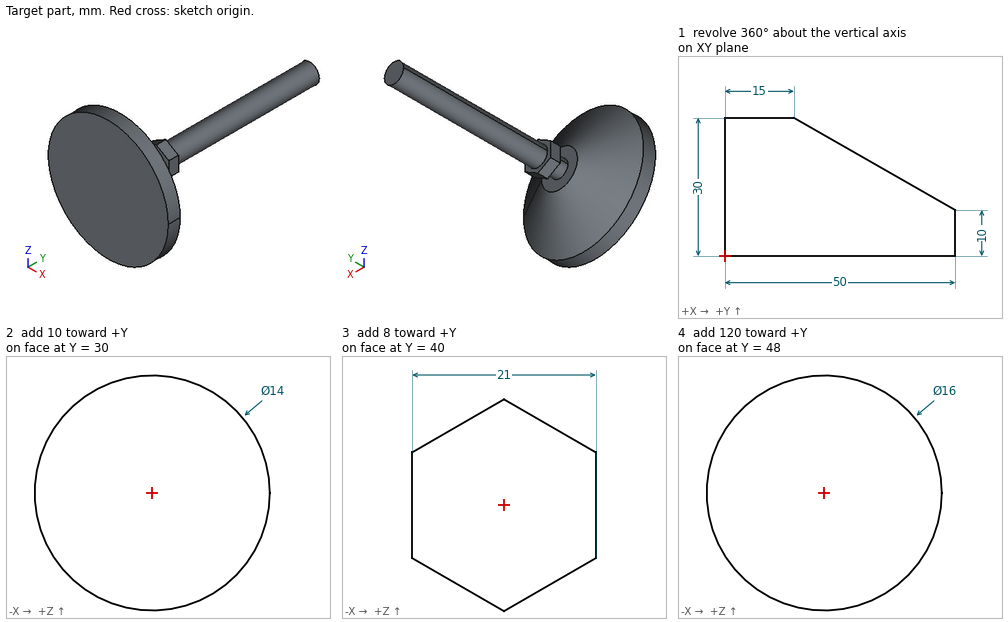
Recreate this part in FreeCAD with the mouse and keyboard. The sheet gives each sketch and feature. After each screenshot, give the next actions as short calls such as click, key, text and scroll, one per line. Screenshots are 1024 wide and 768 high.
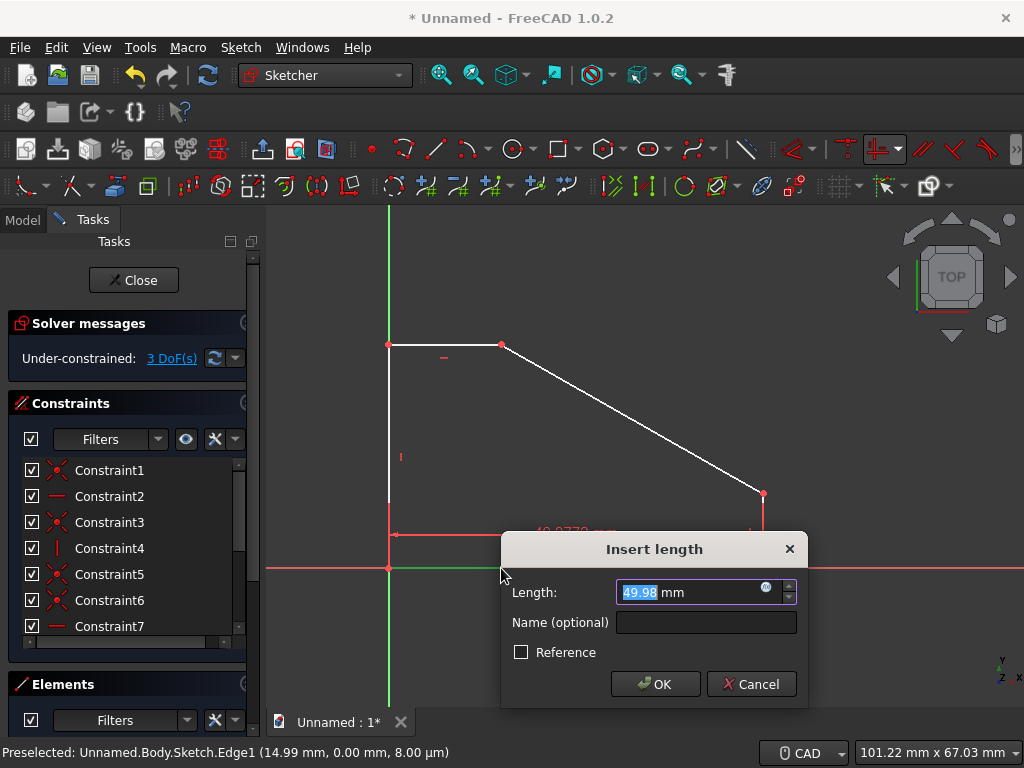
text(50)
key(Return)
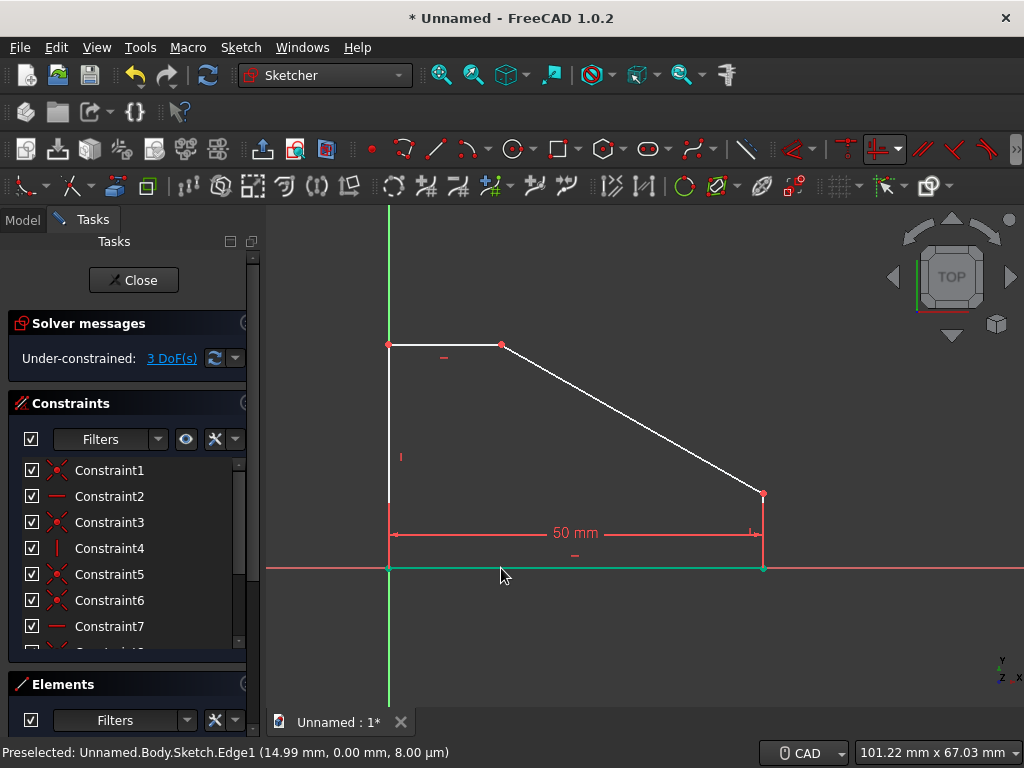
click(763, 546)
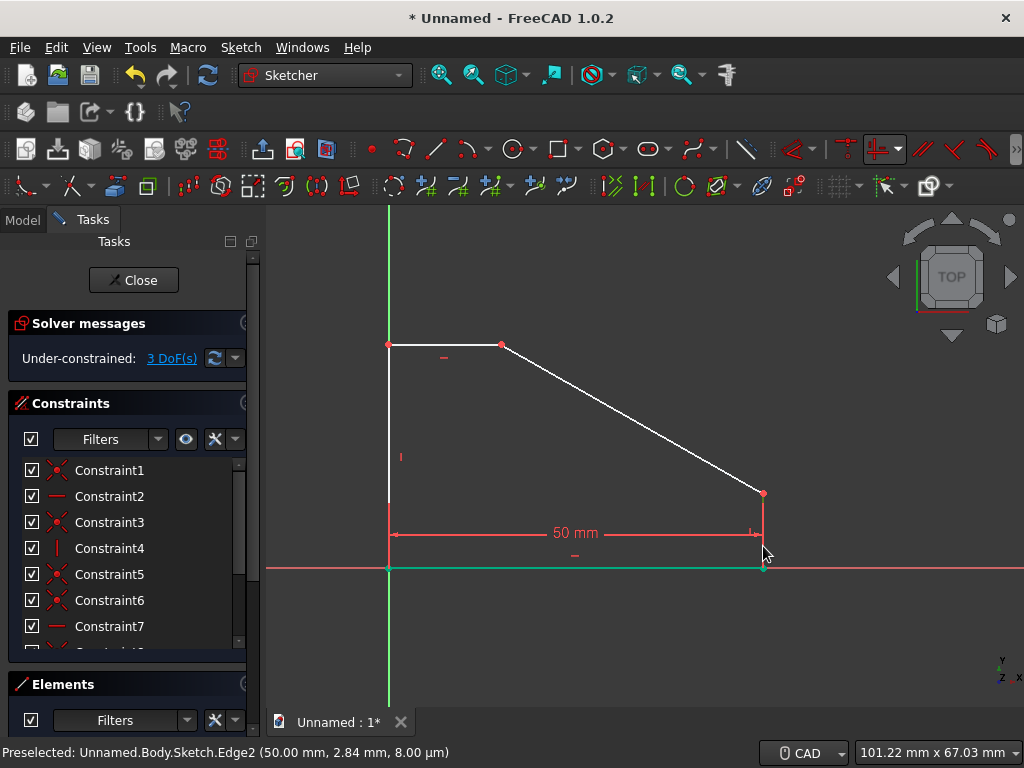
key(i)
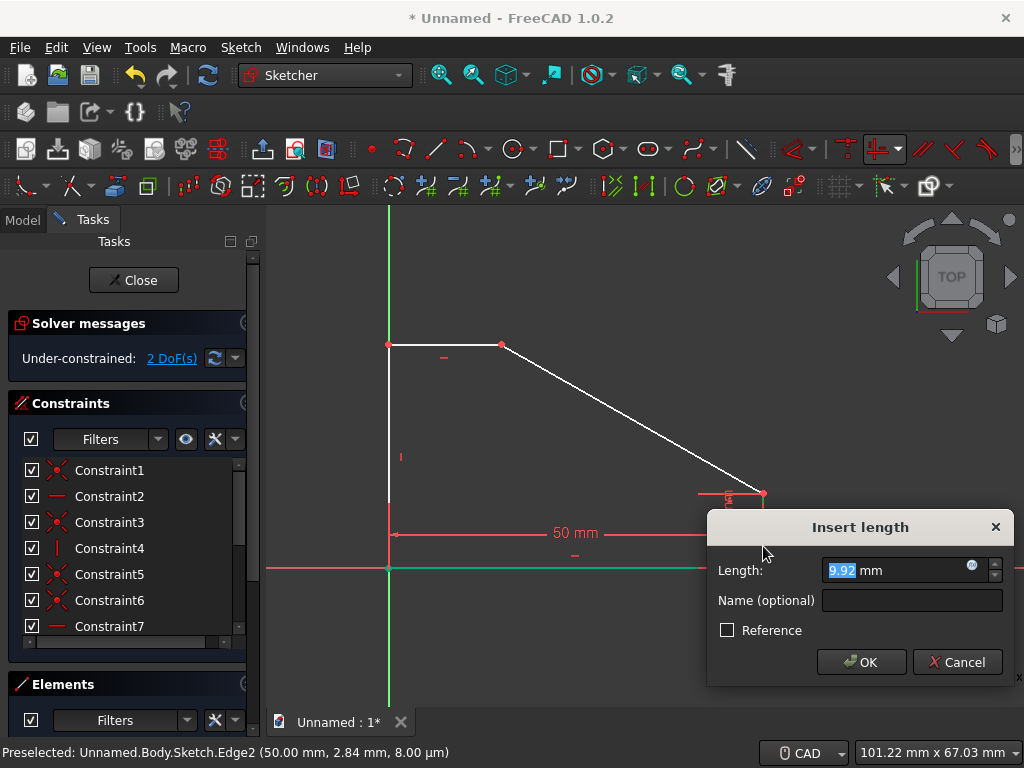
text(10)
key(Return)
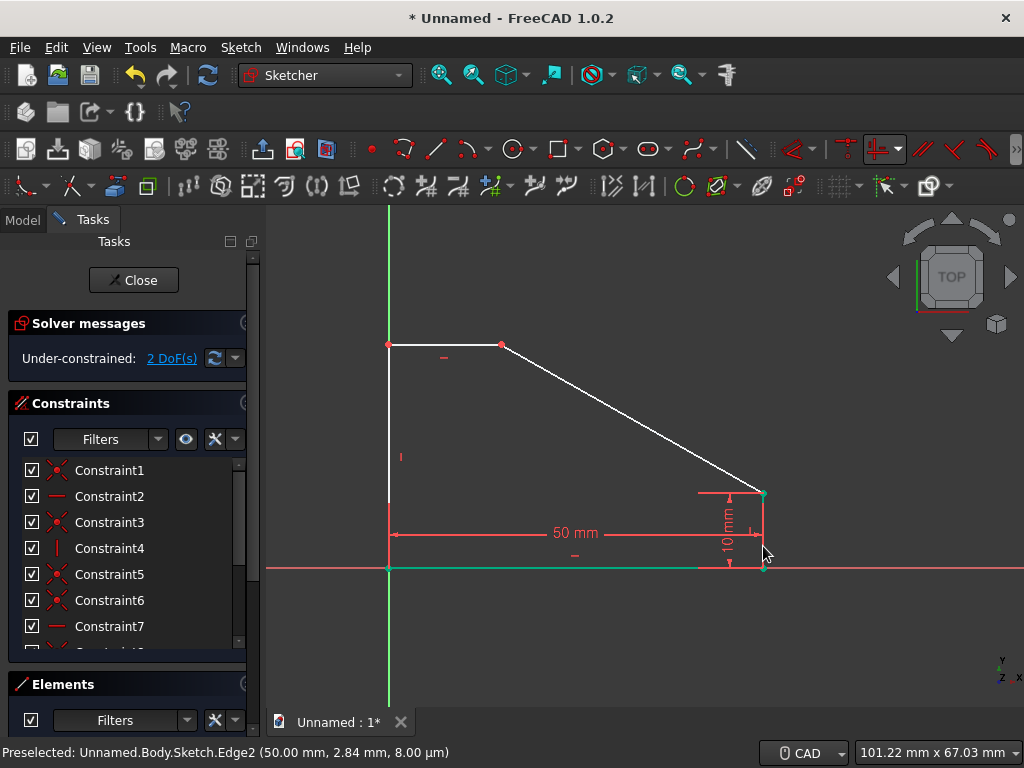
click(467, 345)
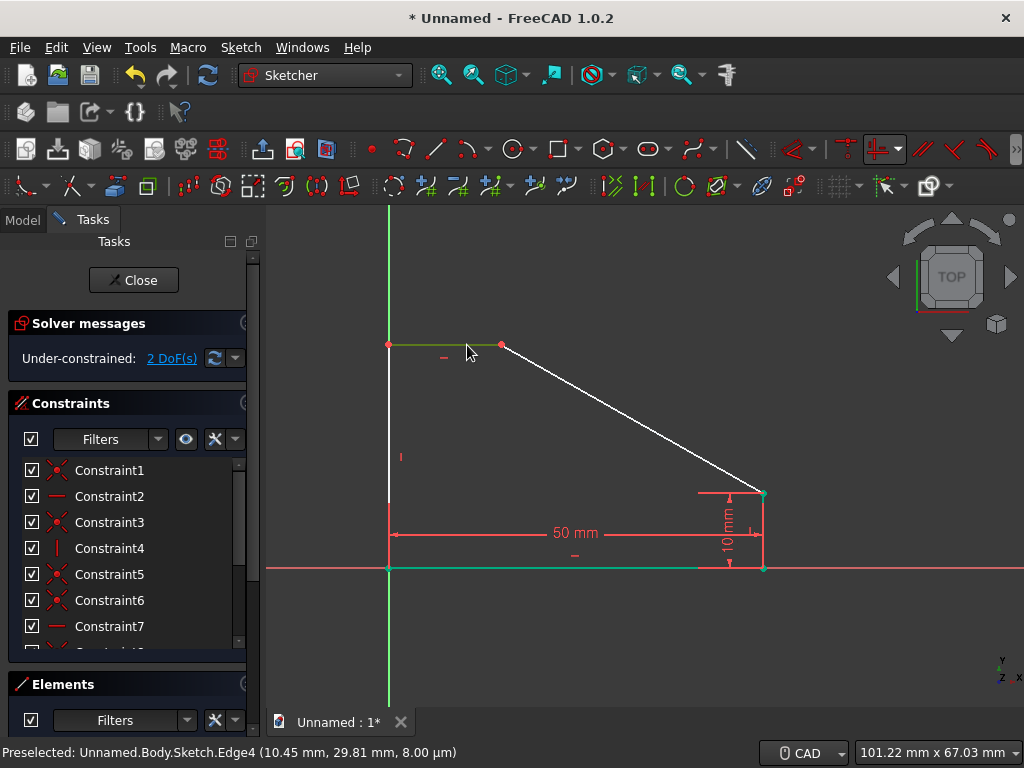
click(814, 150)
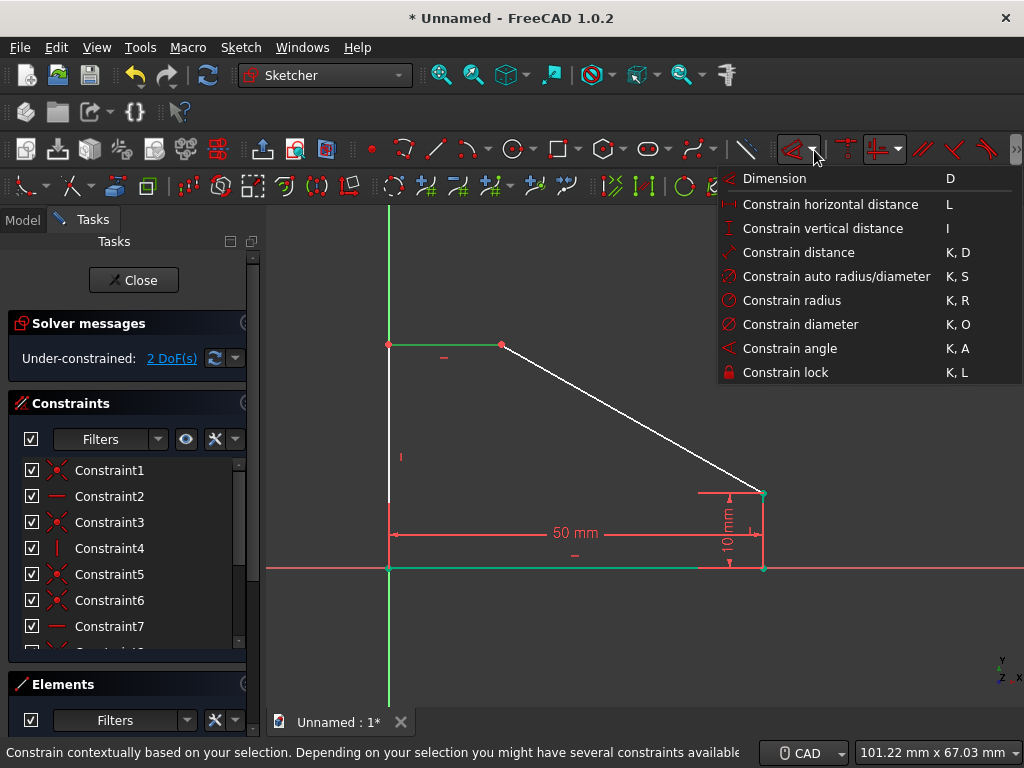
click(870, 204)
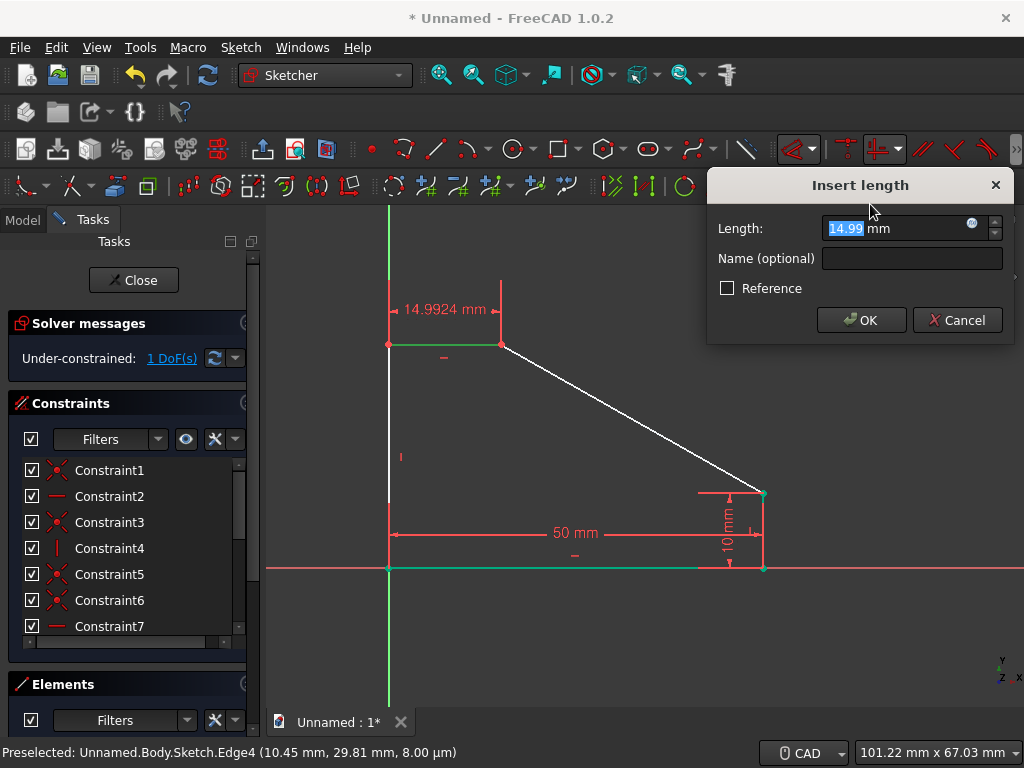
text(15)
key(Return)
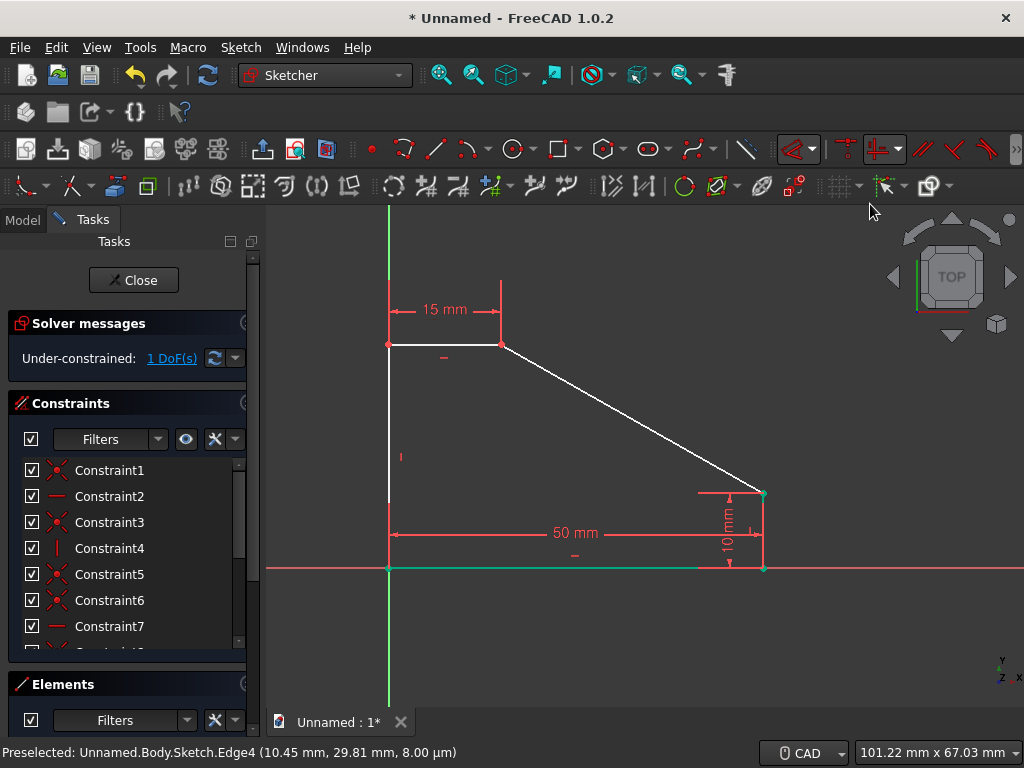
click(389, 412)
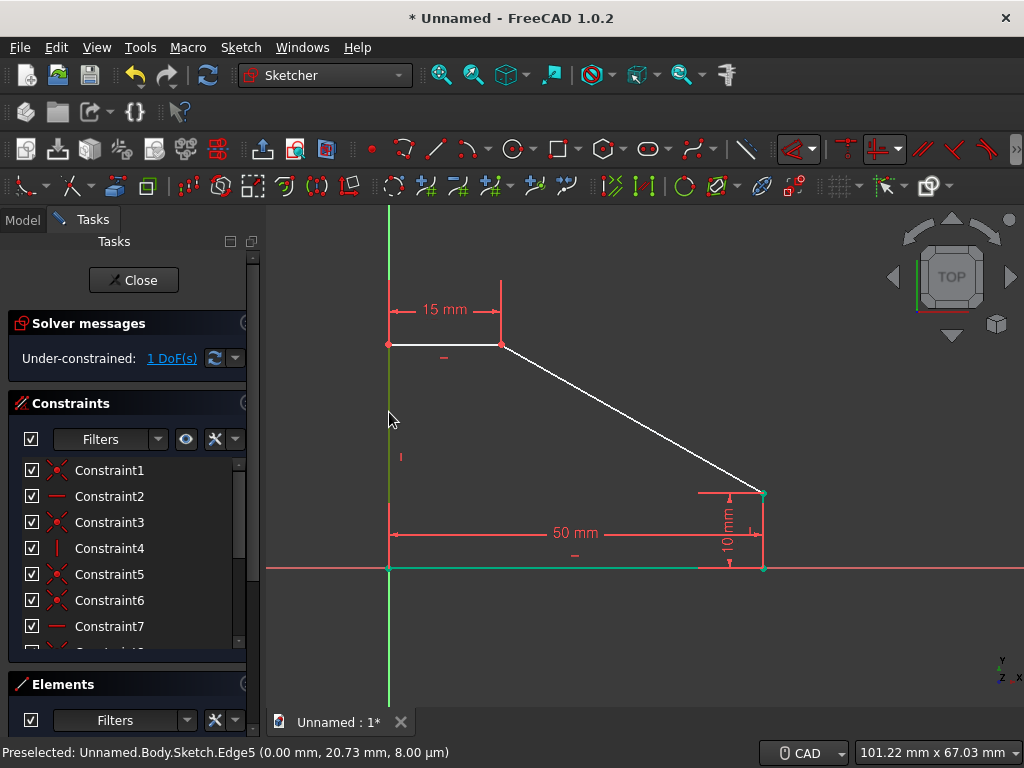
click(814, 150)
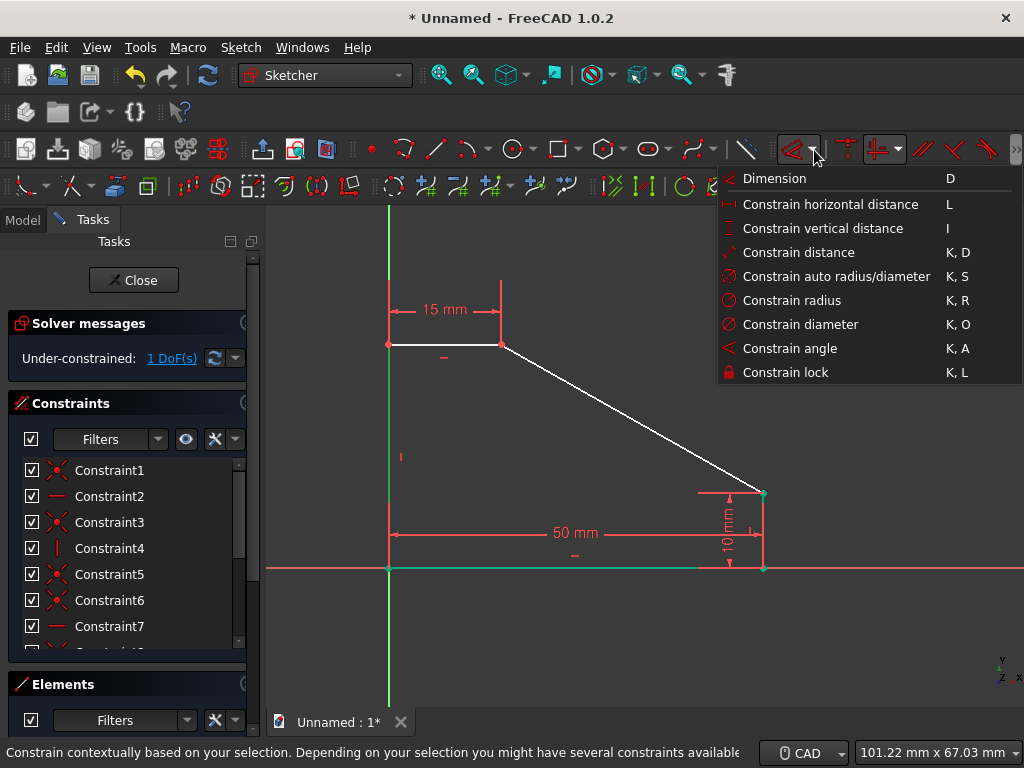
click(870, 228)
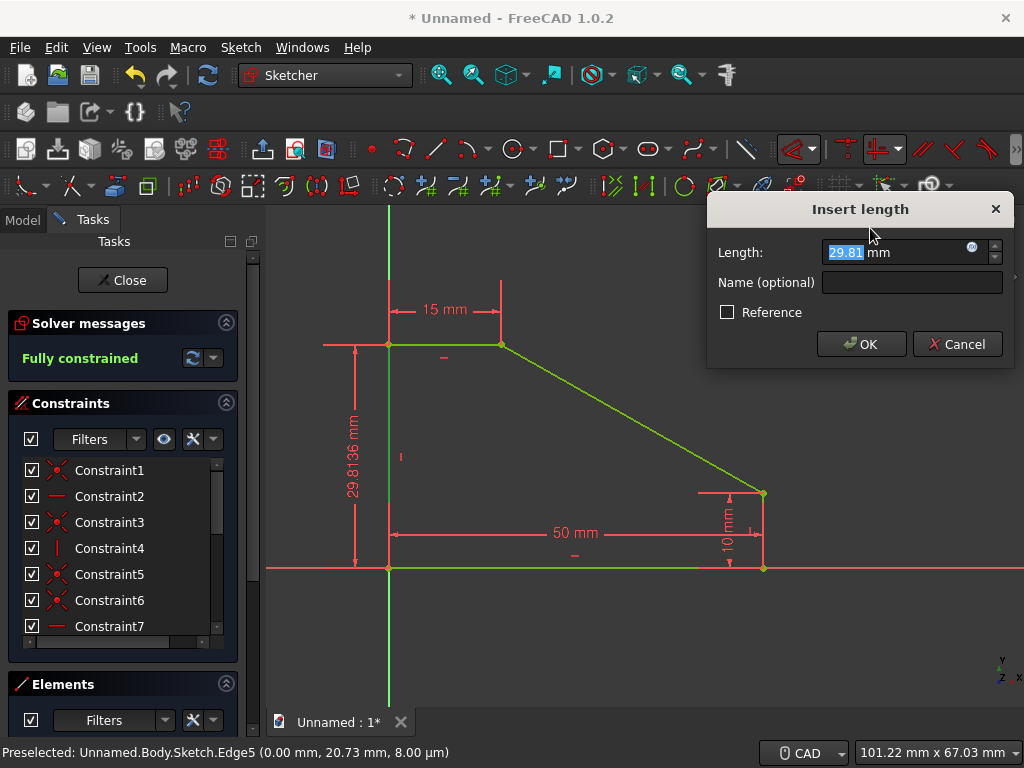
text(30)
key(Return)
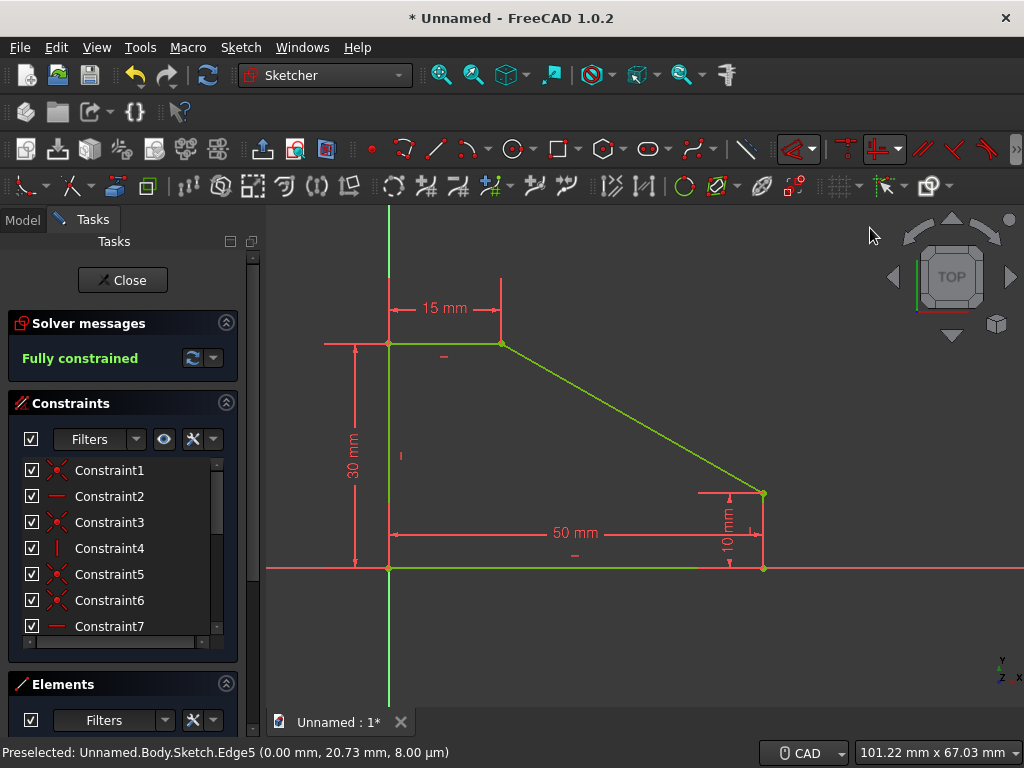
click(123, 280)